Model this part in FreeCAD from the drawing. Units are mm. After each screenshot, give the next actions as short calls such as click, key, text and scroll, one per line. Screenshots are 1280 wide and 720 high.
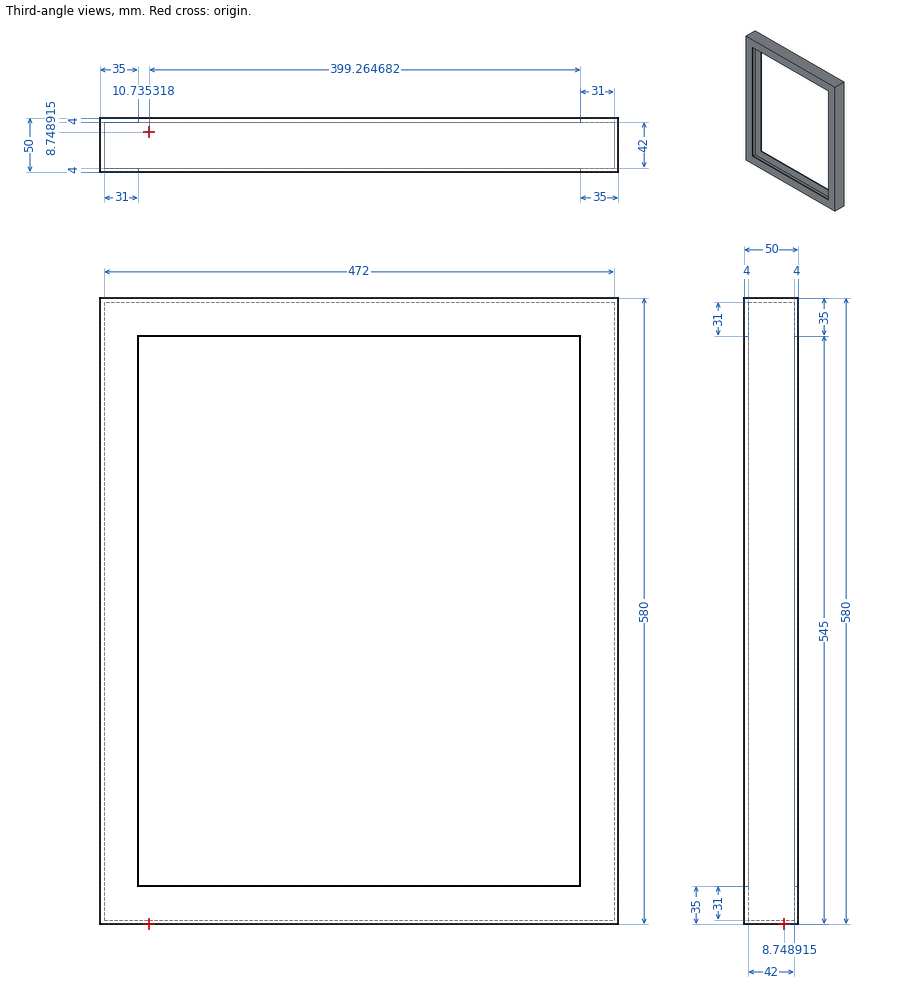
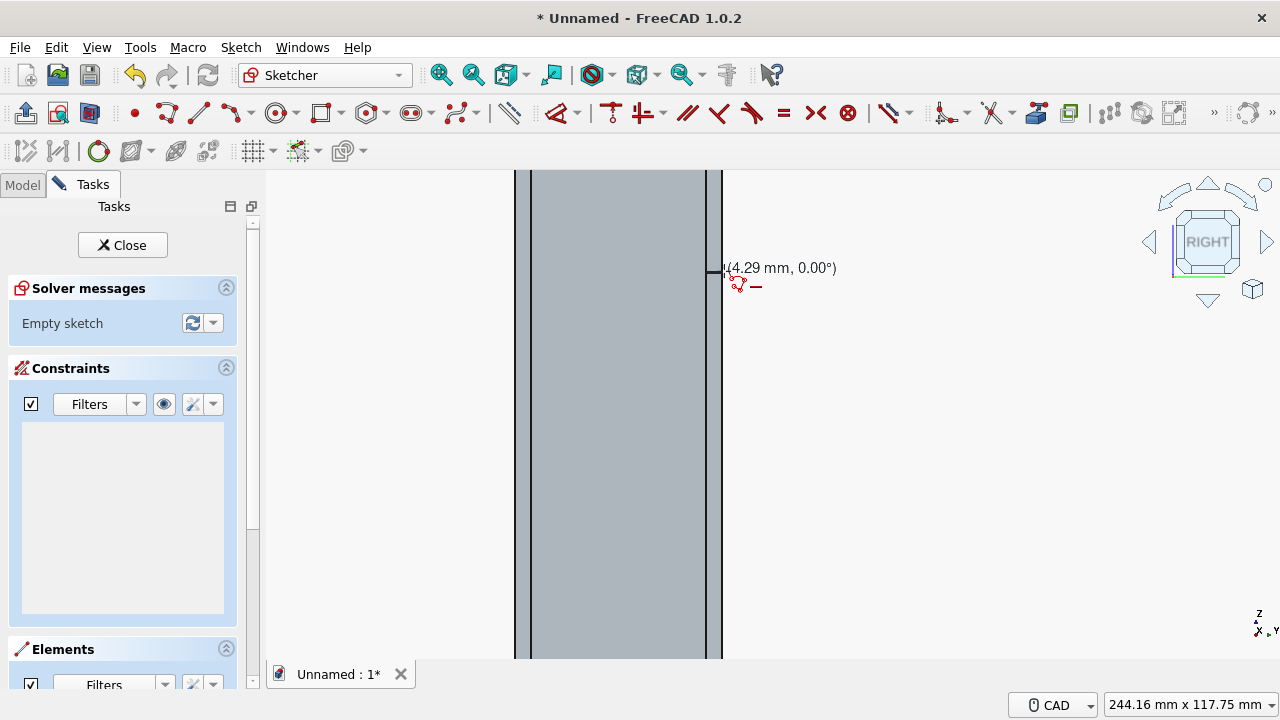
click(722, 271)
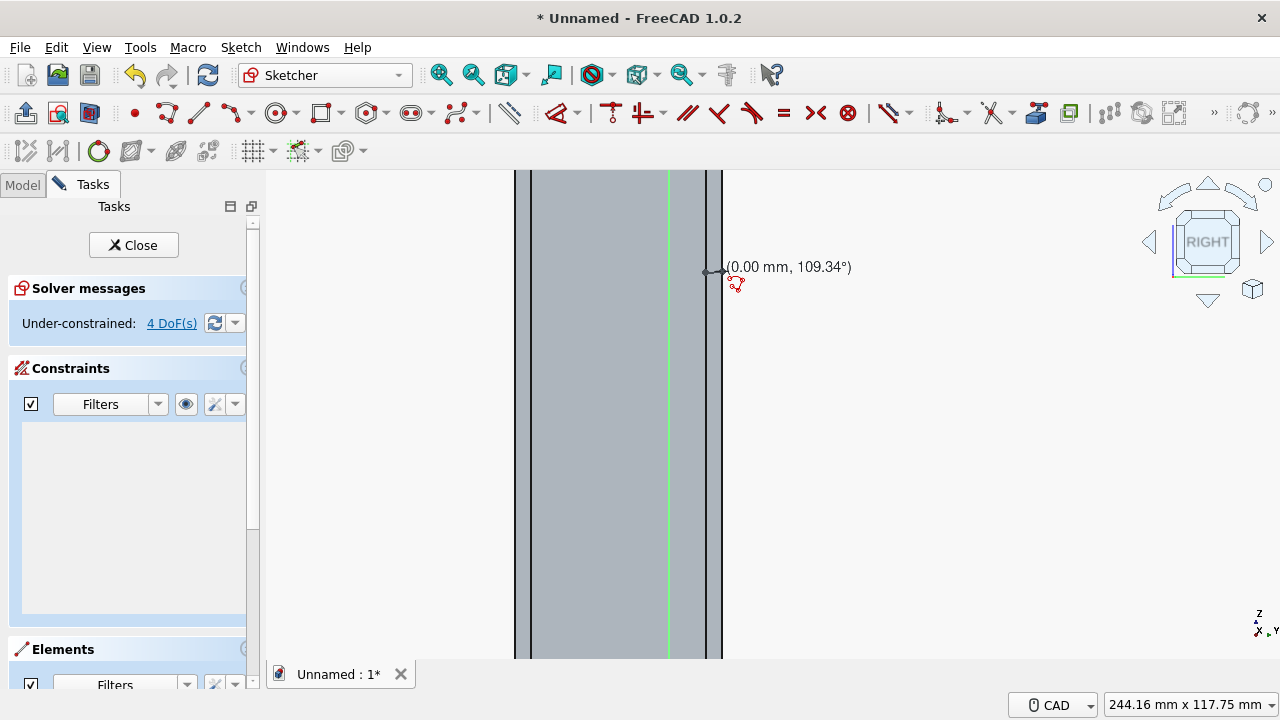
scroll(718, 271, down, 10)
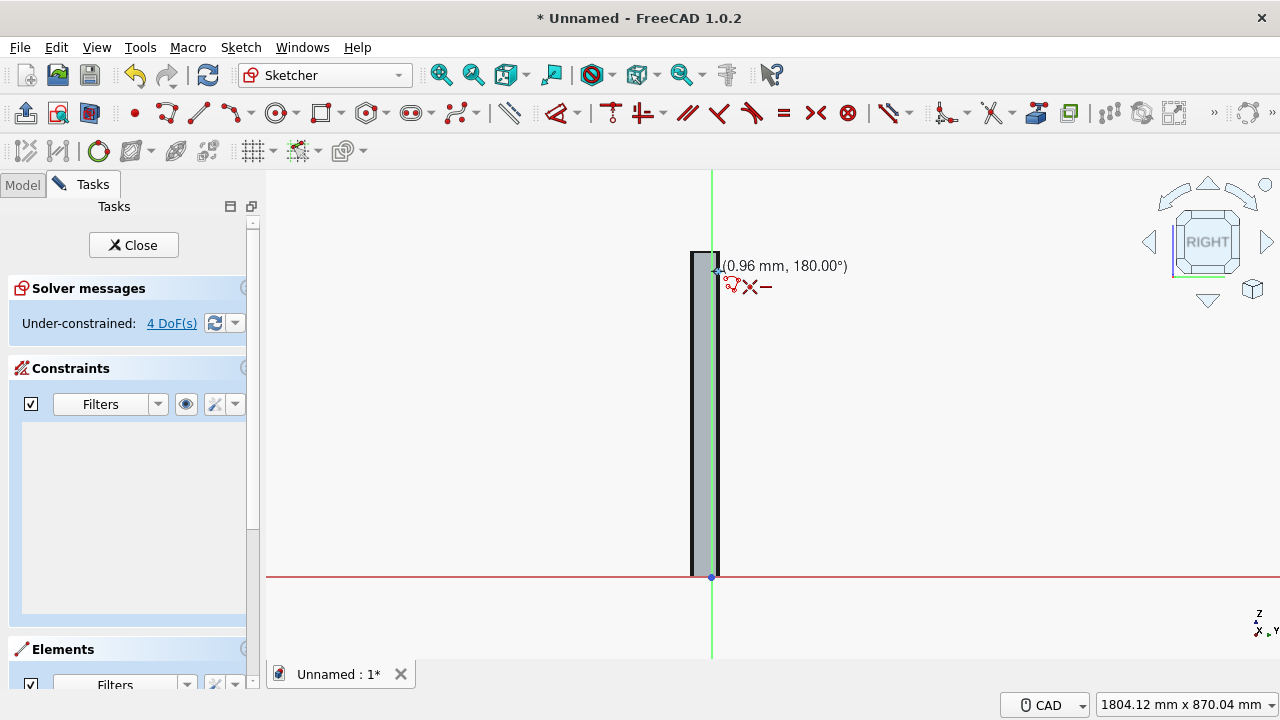
scroll(719, 252, up, 4)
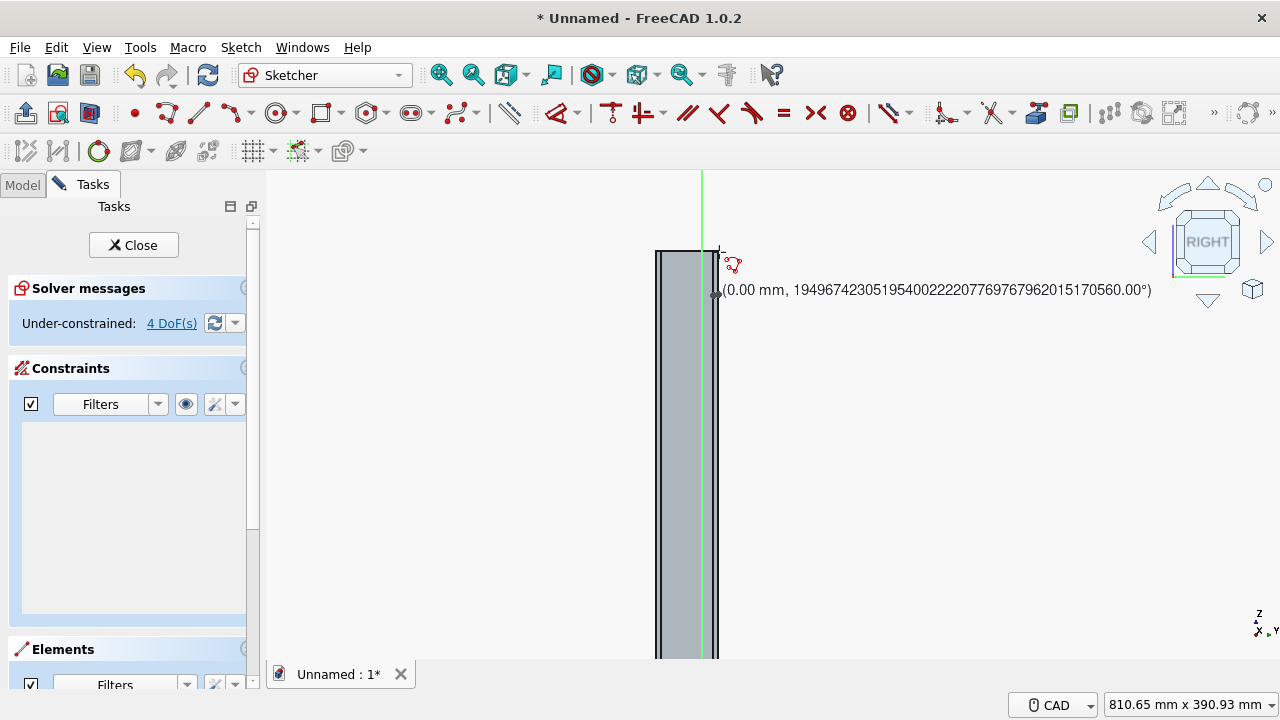
click(718, 251)
click(656, 251)
click(656, 294)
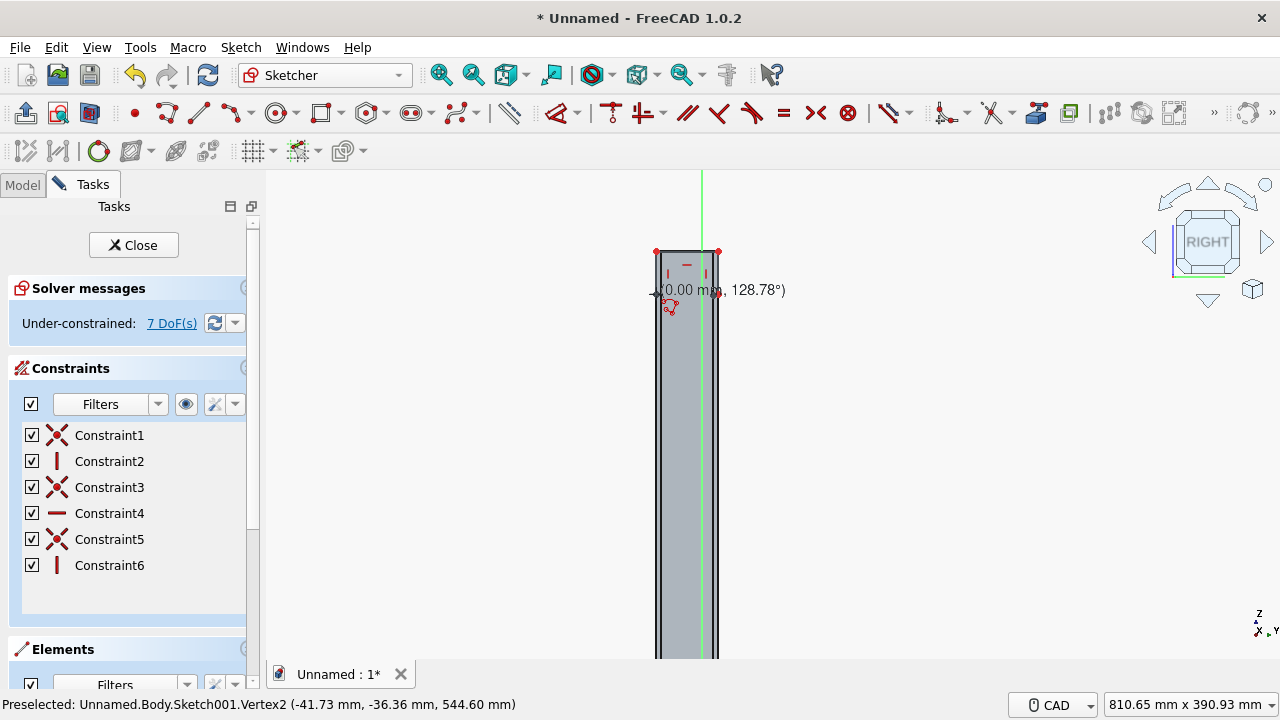
scroll(661, 294, up, 6)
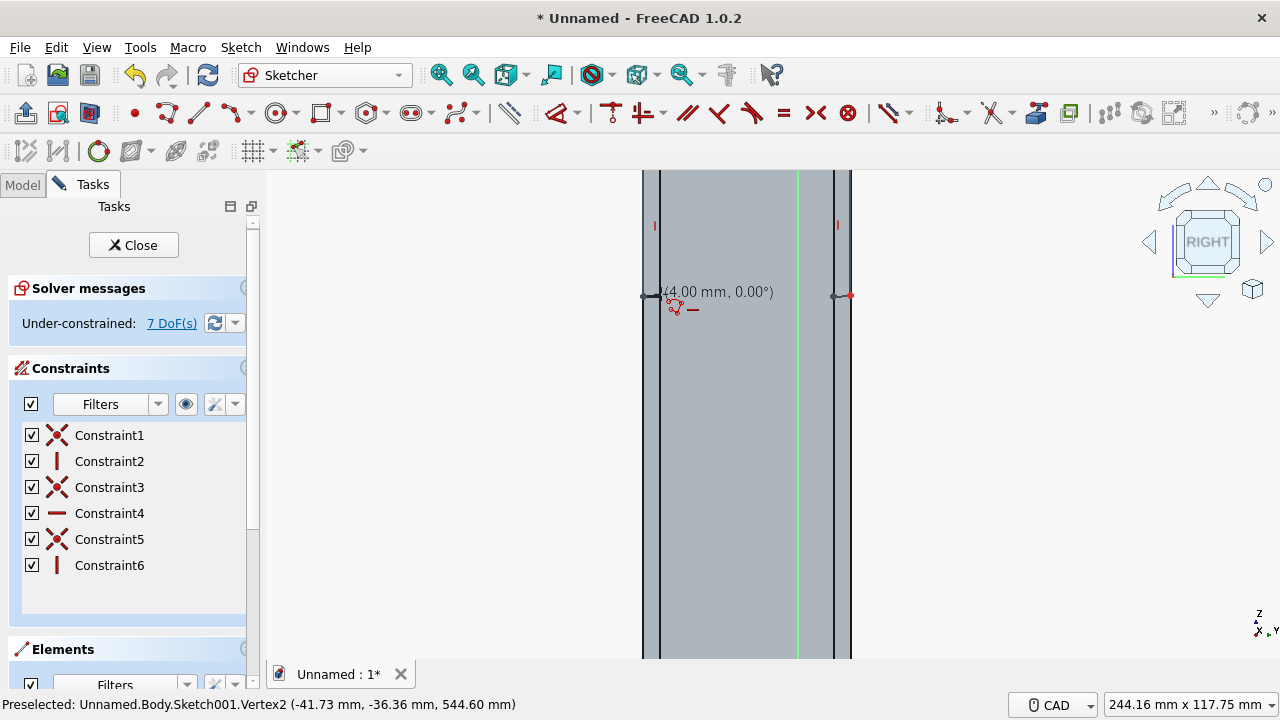
click(660, 293)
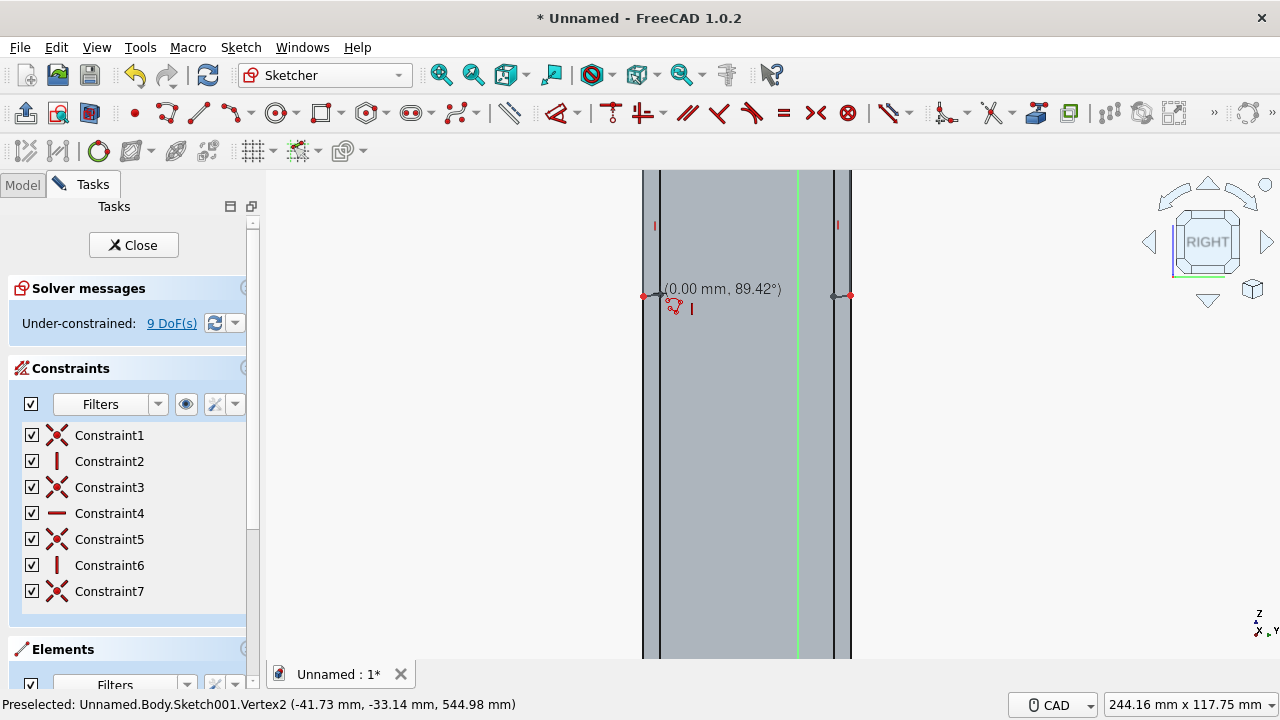
scroll(698, 267, down, 10)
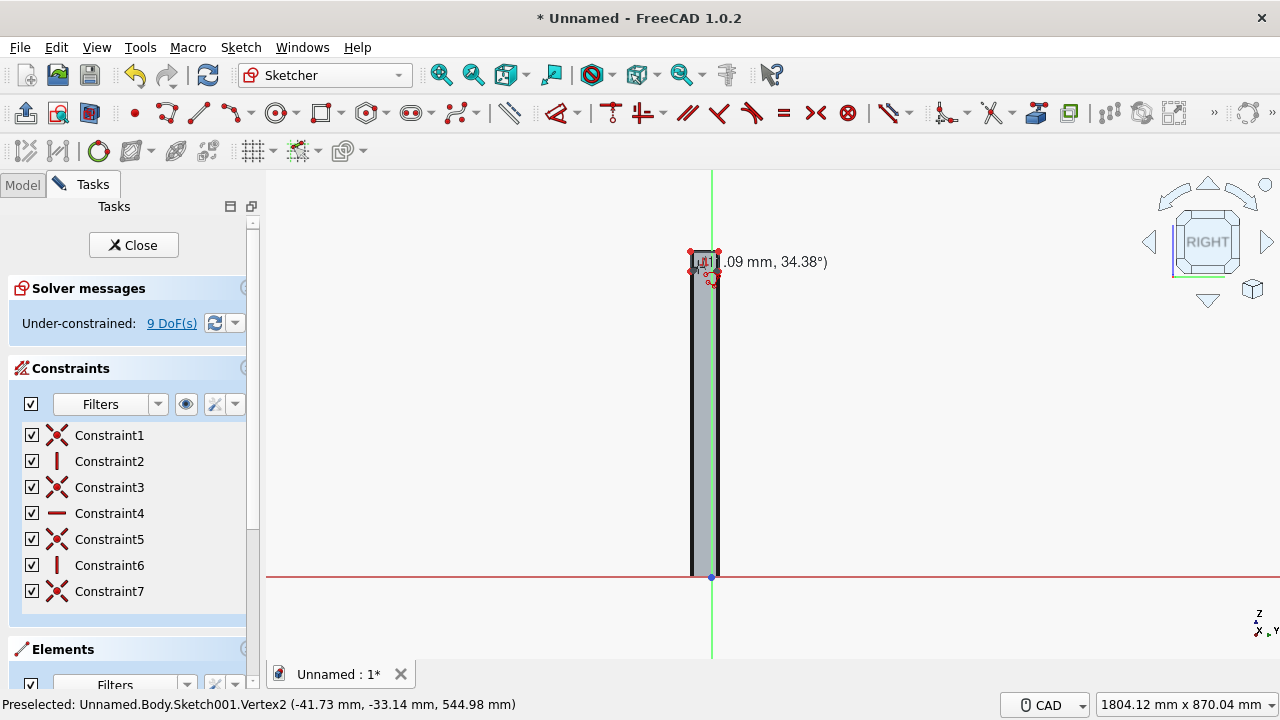
scroll(693, 254, up, 10)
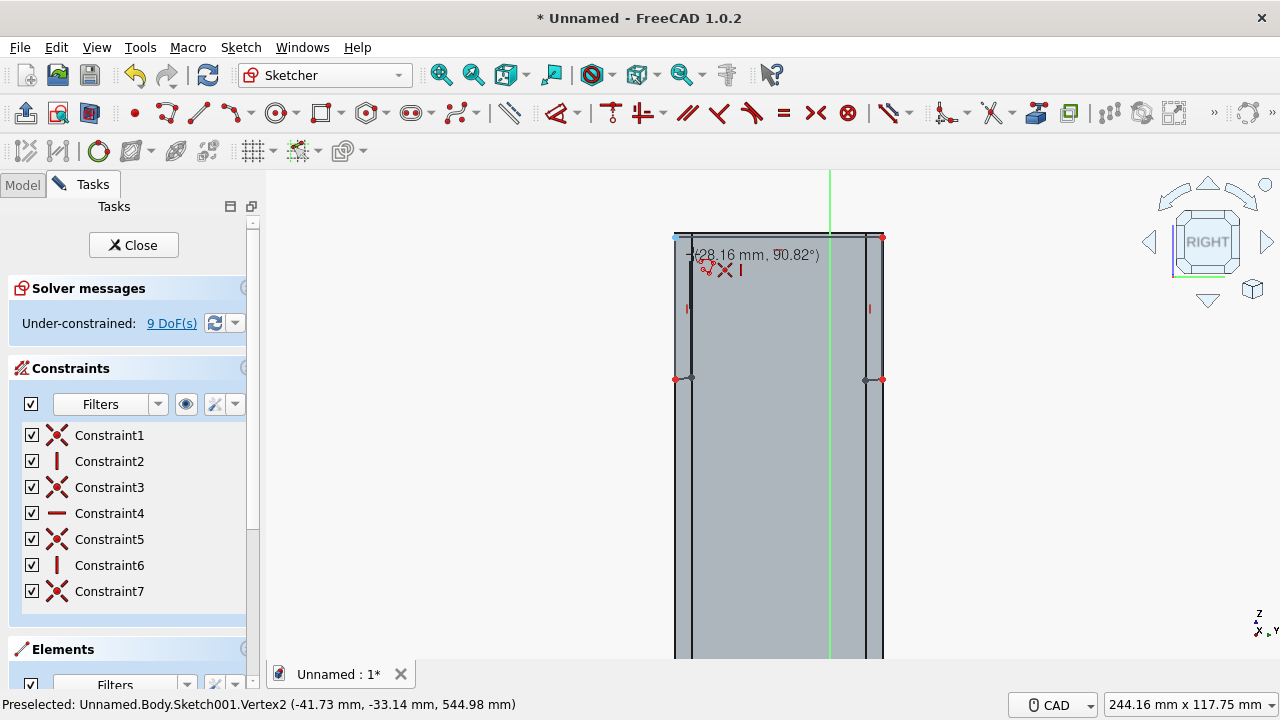
click(692, 249)
click(866, 249)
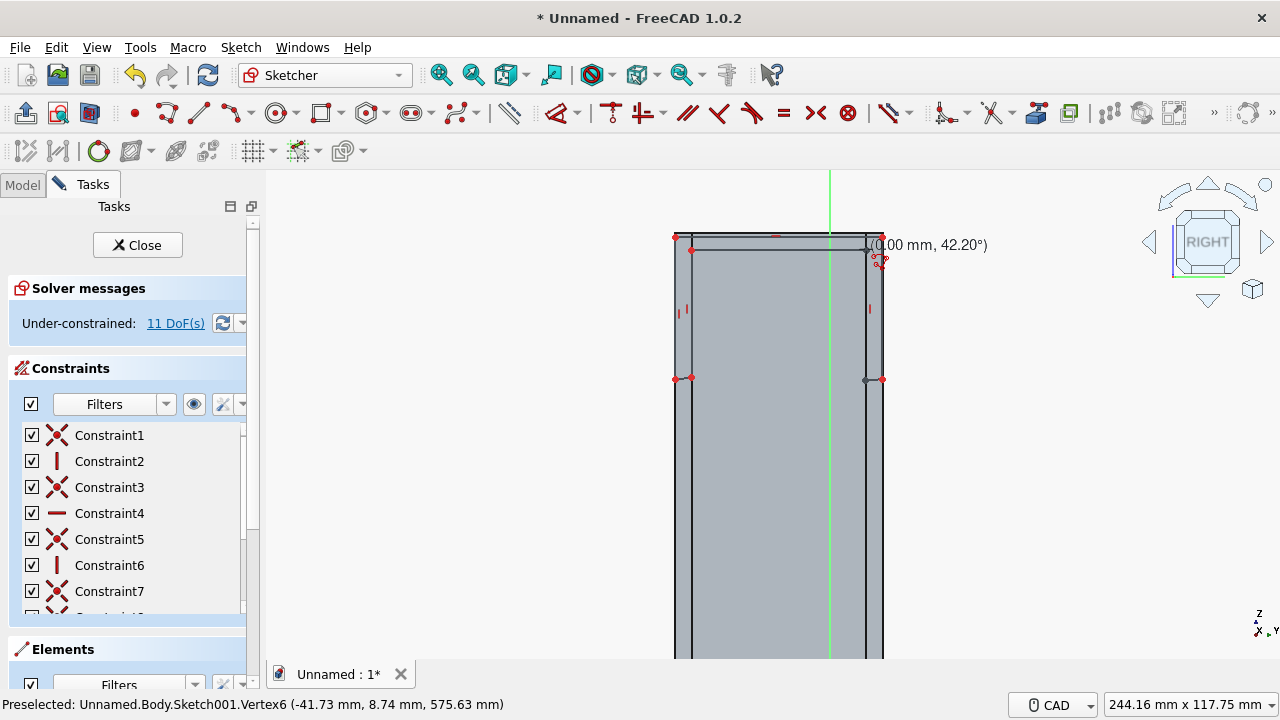
scroll(866, 378, up, 4)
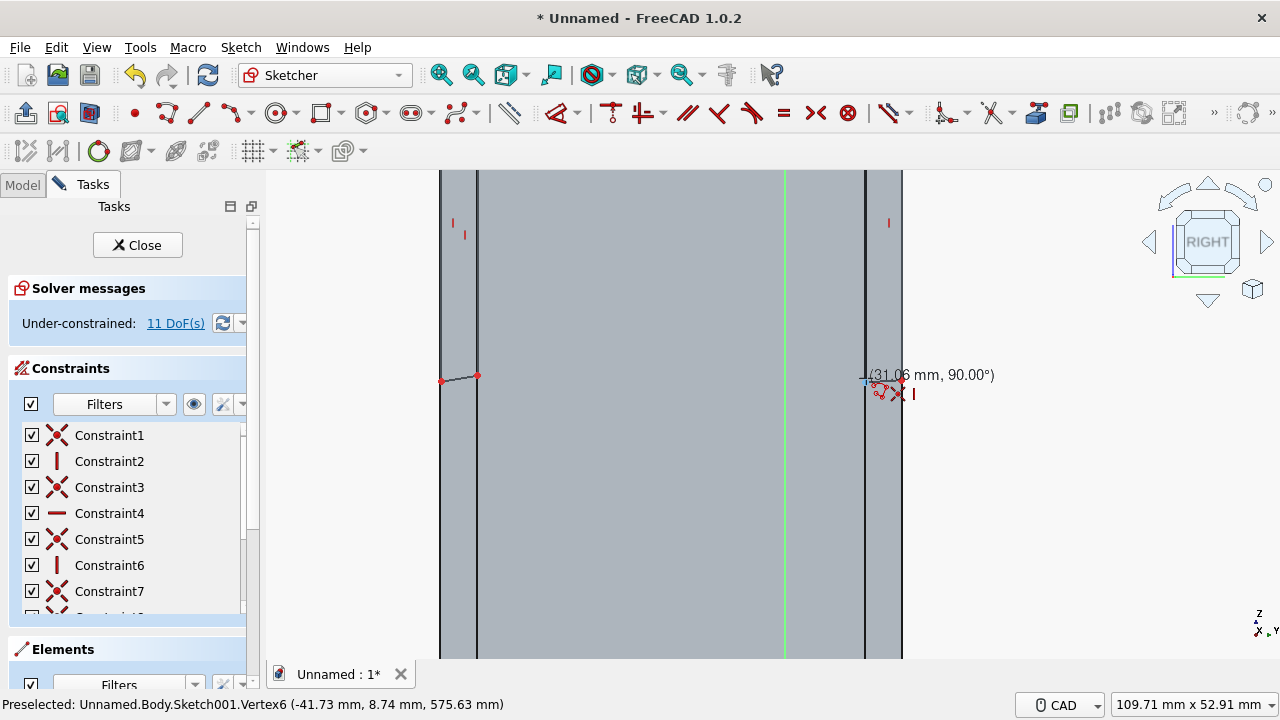
click(865, 382)